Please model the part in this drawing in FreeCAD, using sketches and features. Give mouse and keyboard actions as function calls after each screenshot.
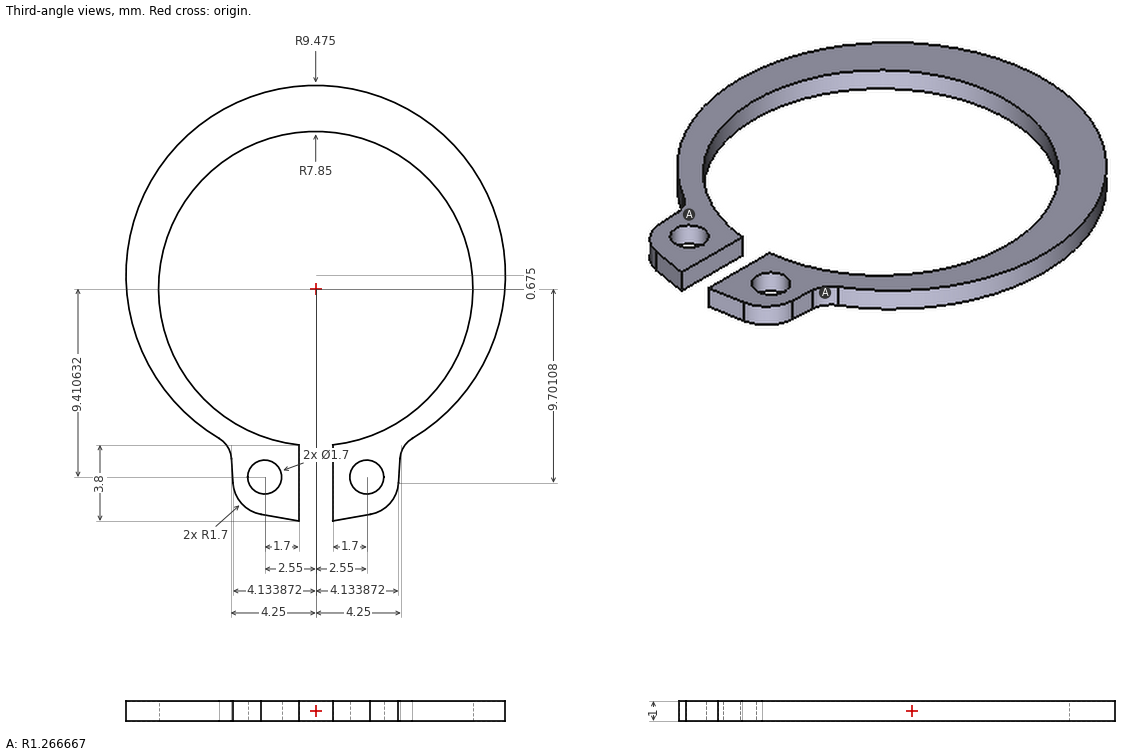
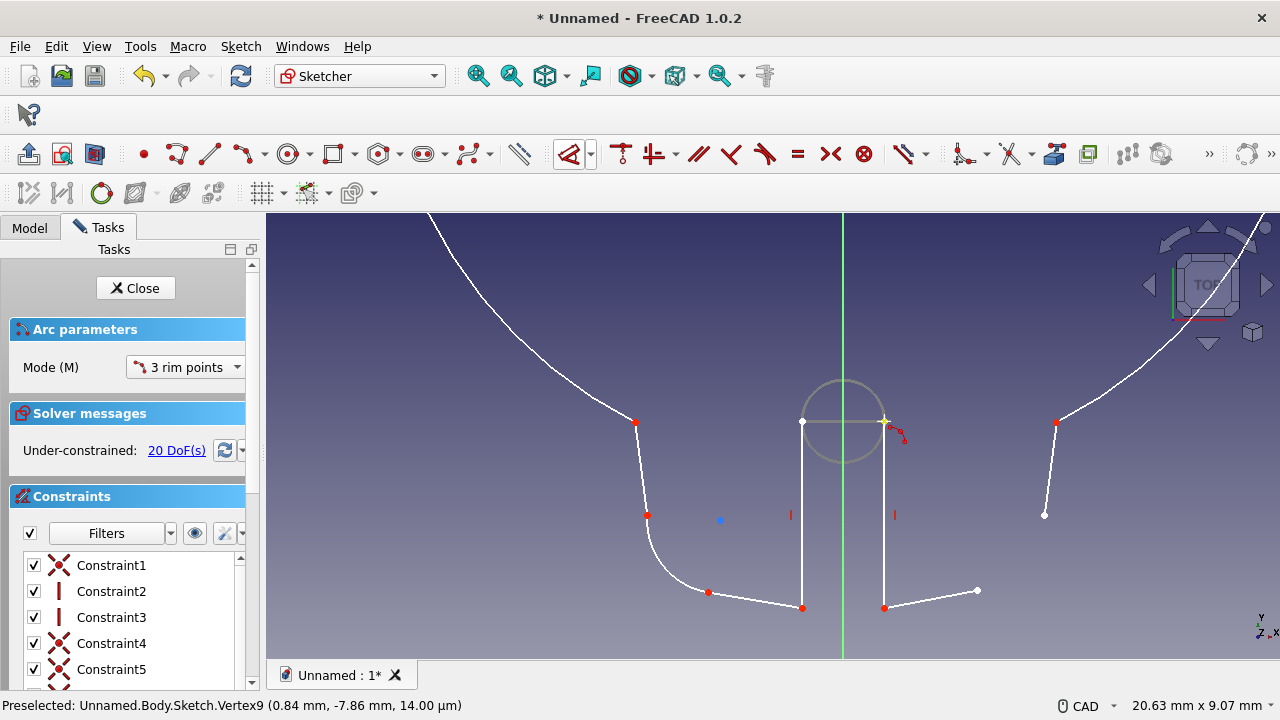
scroll(659, 556, down, 7)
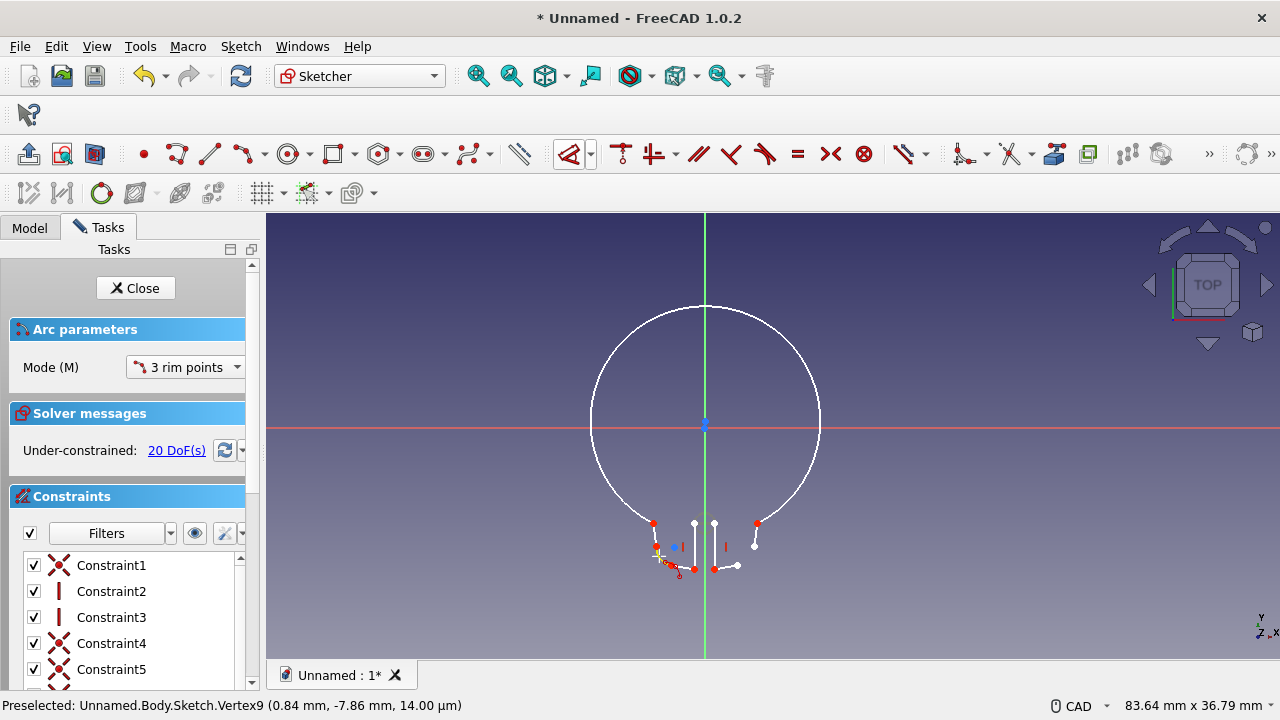
click(759, 350)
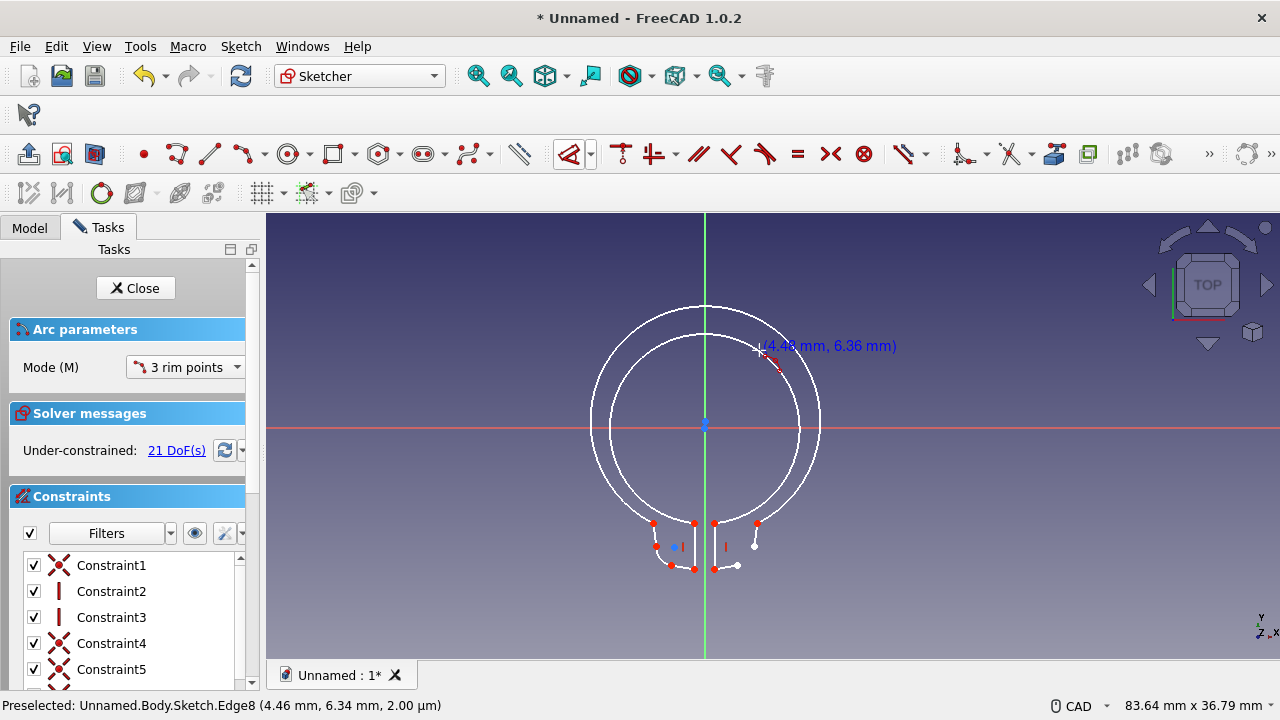
scroll(738, 565, up, 2)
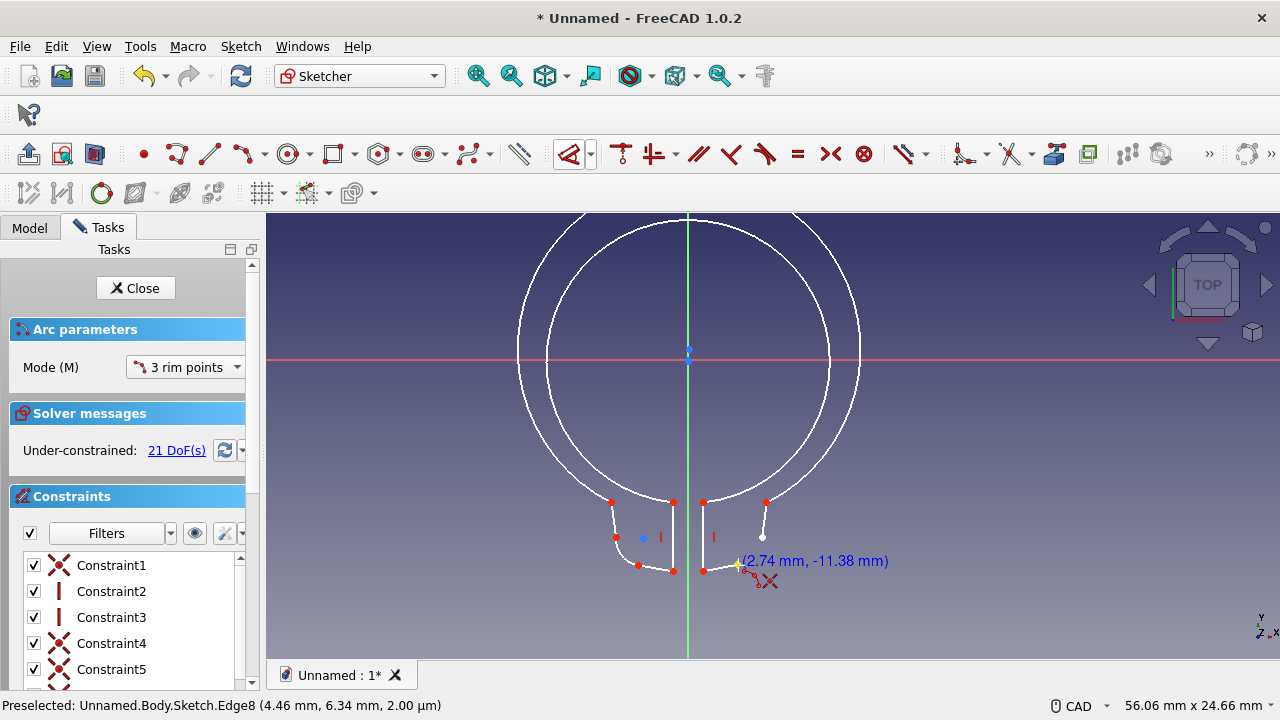
click(738, 565)
click(762, 537)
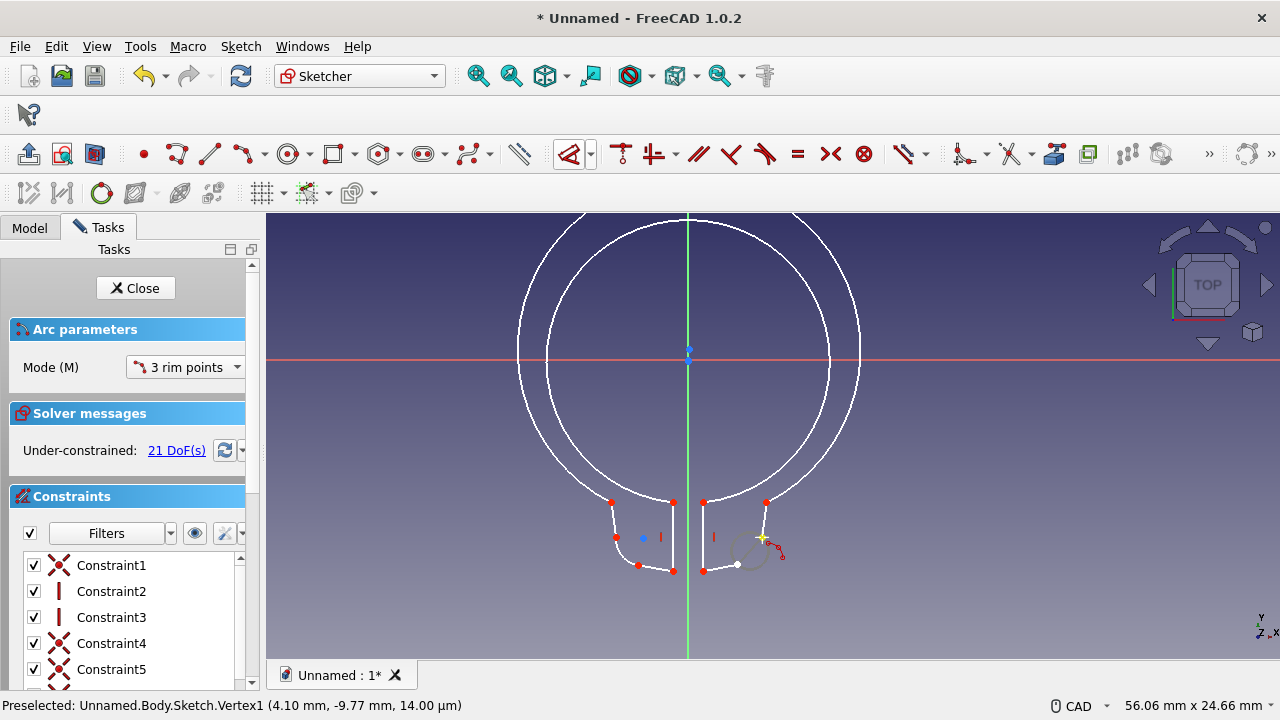
scroll(755, 554, up, 5)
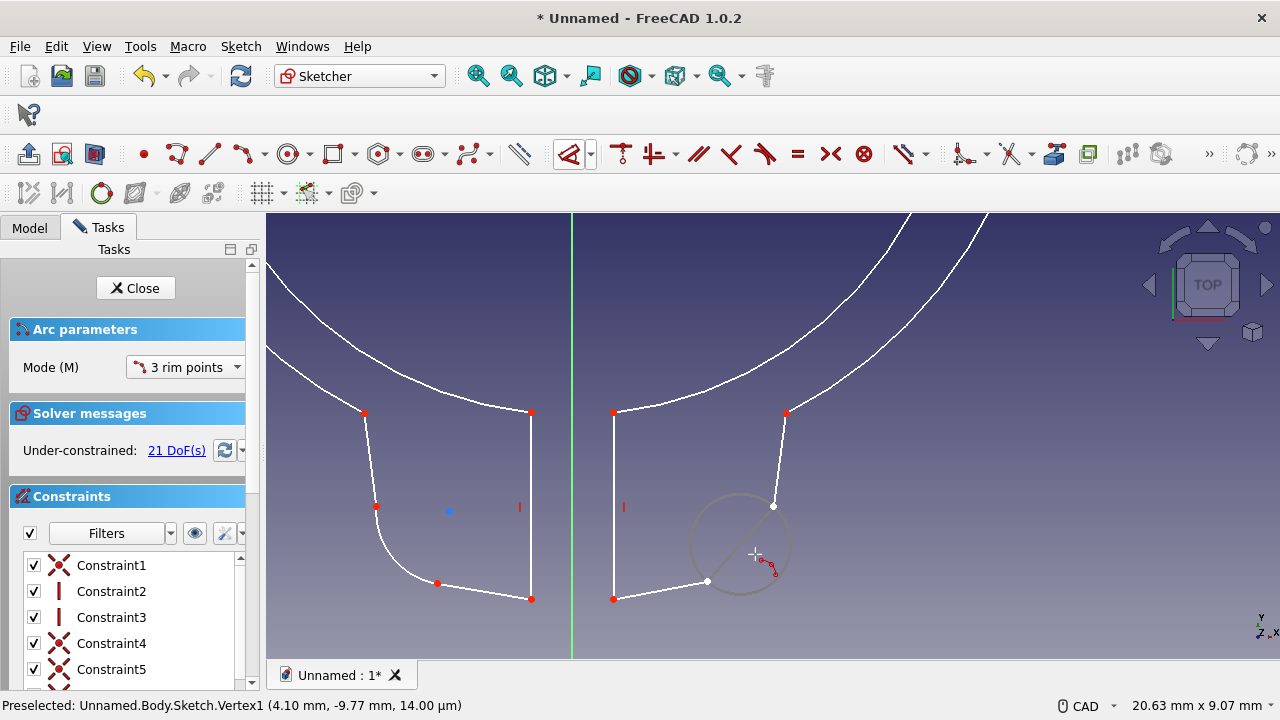
click(755, 554)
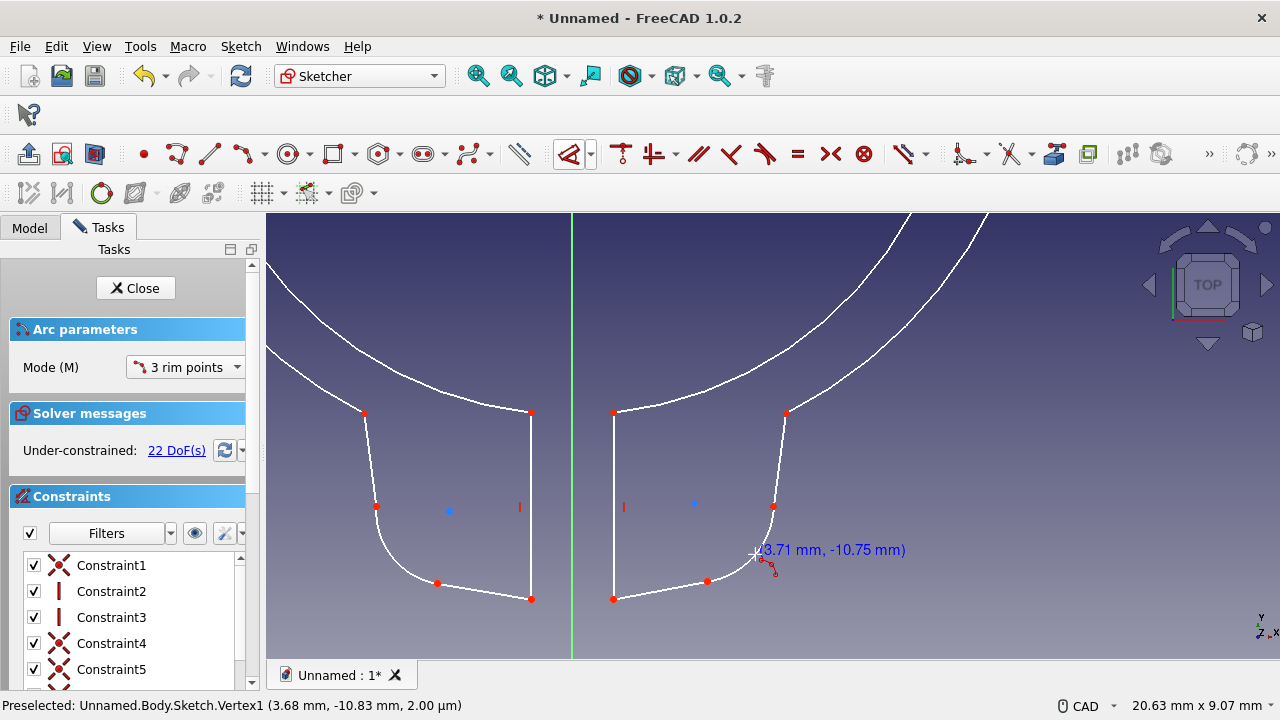
click(288, 154)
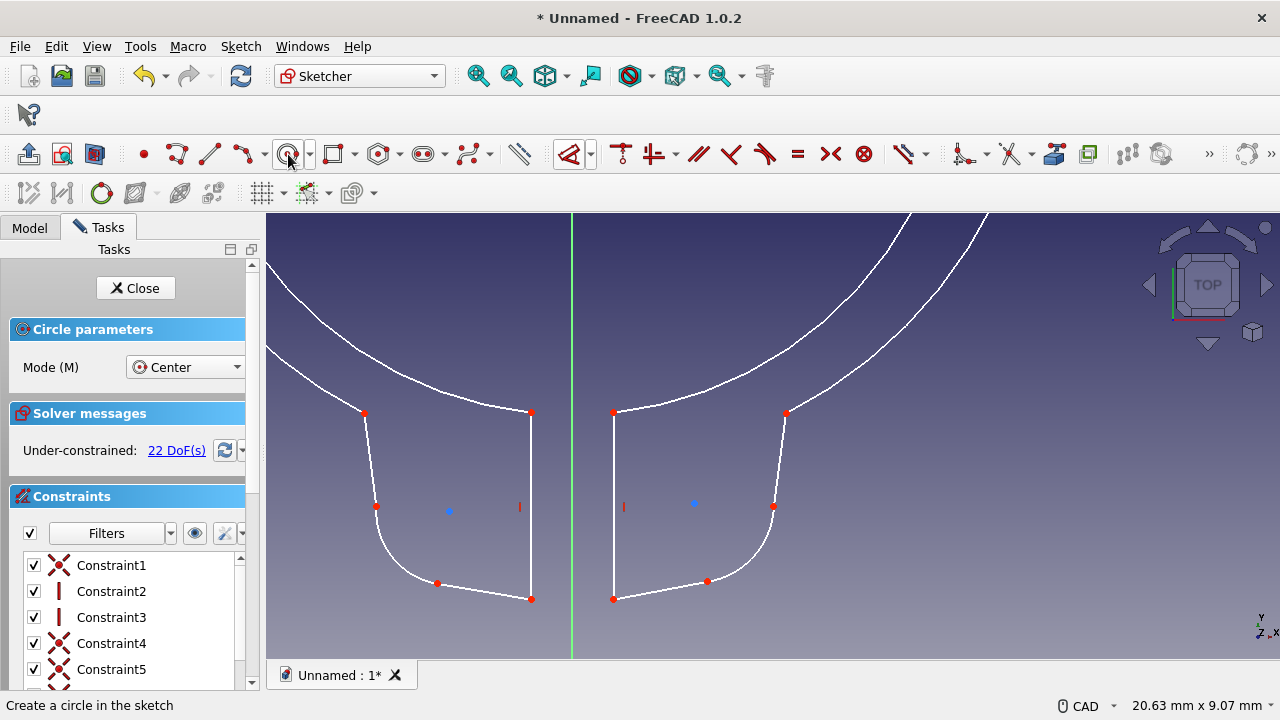
scroll(447, 489, up, 2)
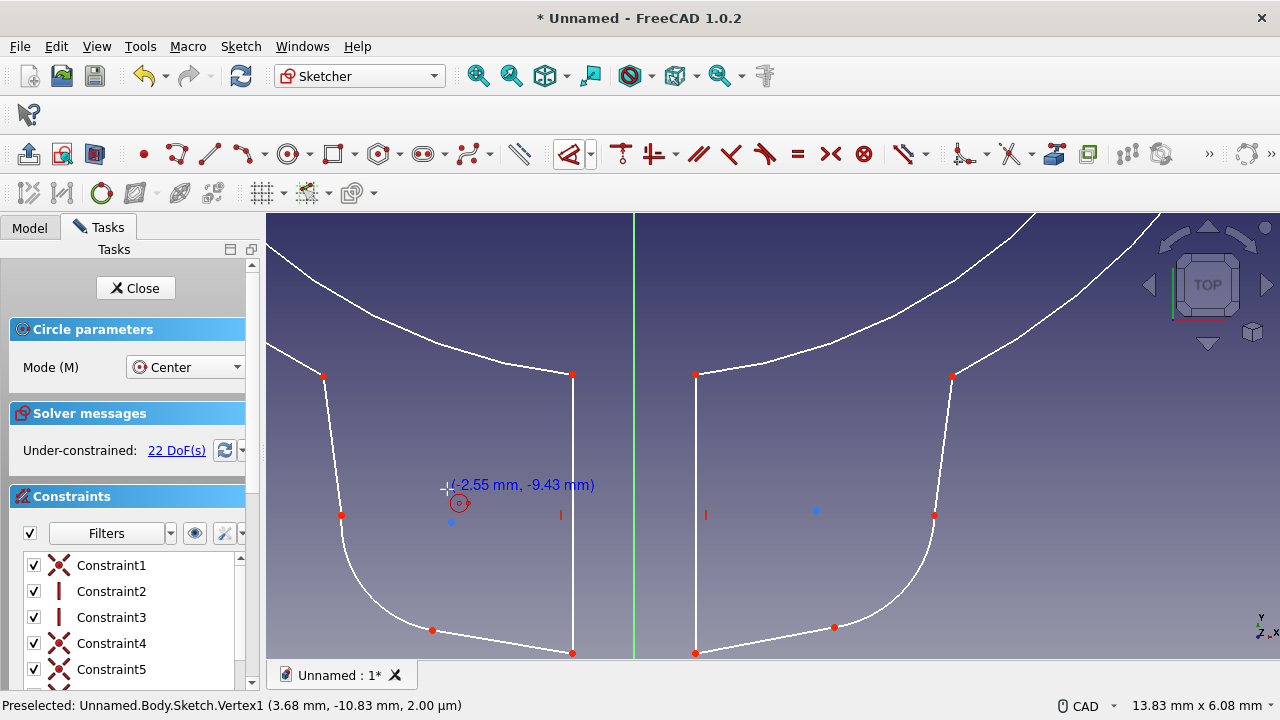
click(447, 489)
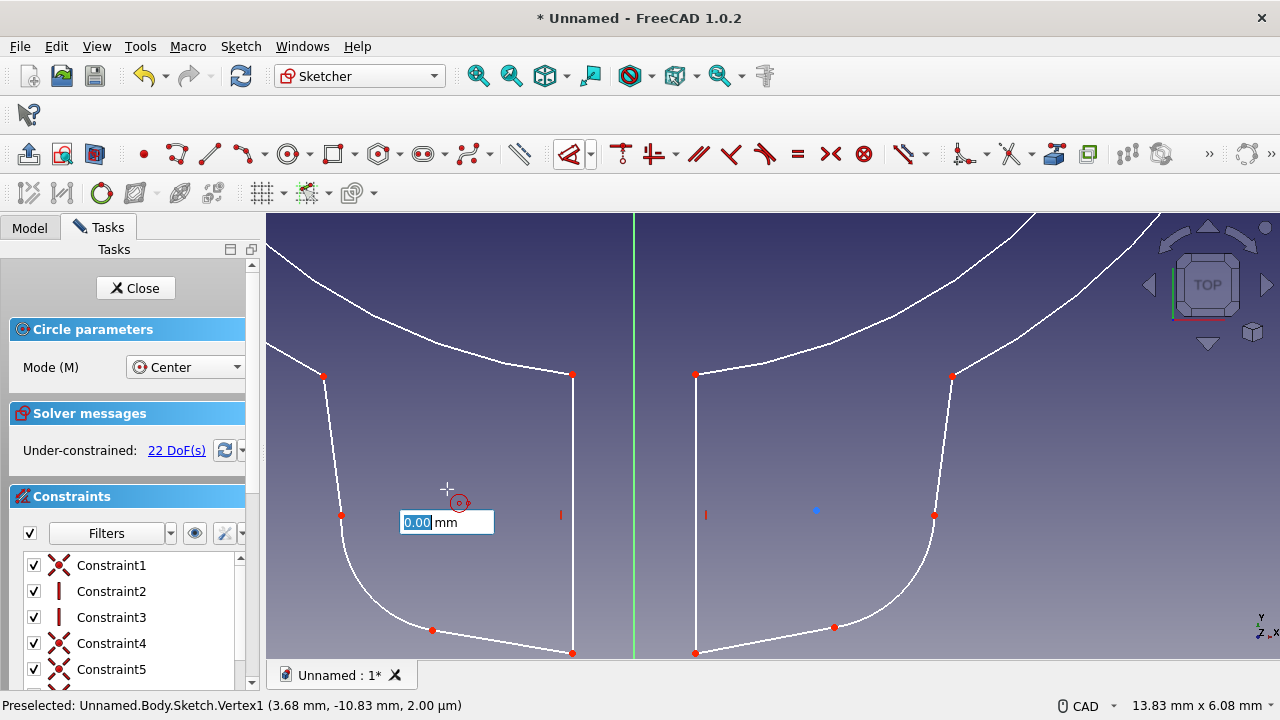
scroll(718, 552, down, 9)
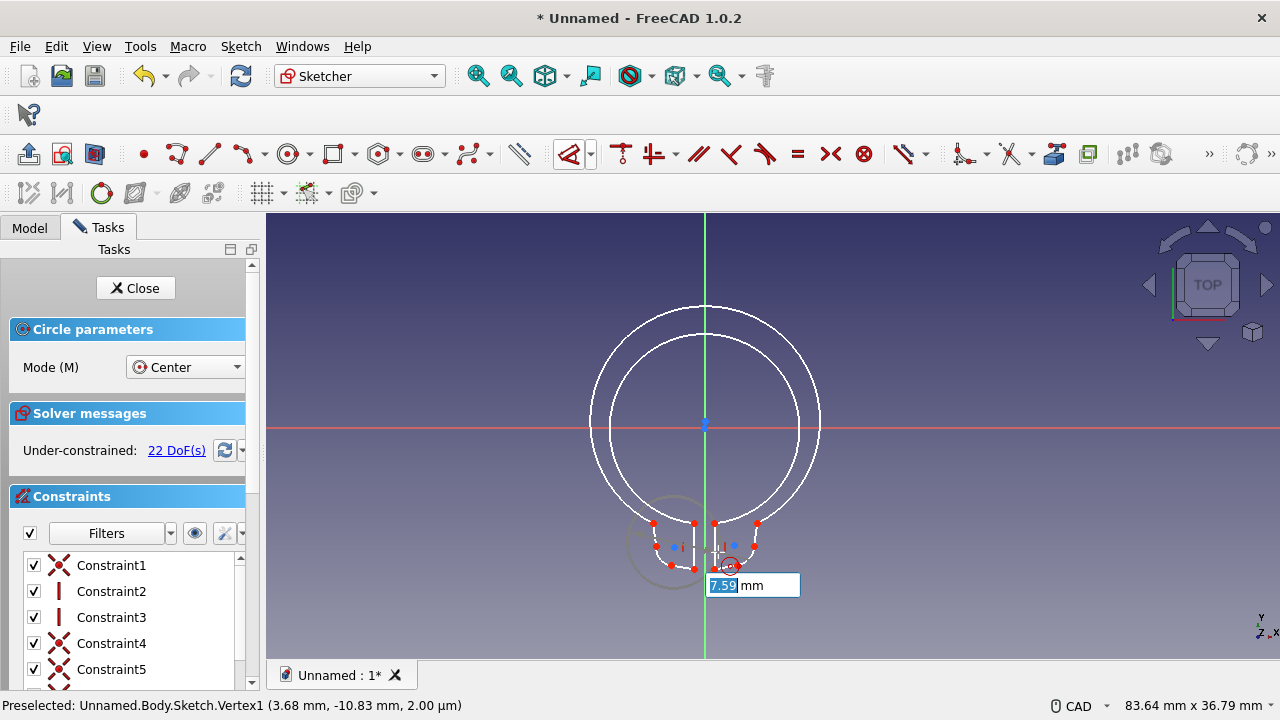
scroll(681, 535, up, 2)
move(681, 534)